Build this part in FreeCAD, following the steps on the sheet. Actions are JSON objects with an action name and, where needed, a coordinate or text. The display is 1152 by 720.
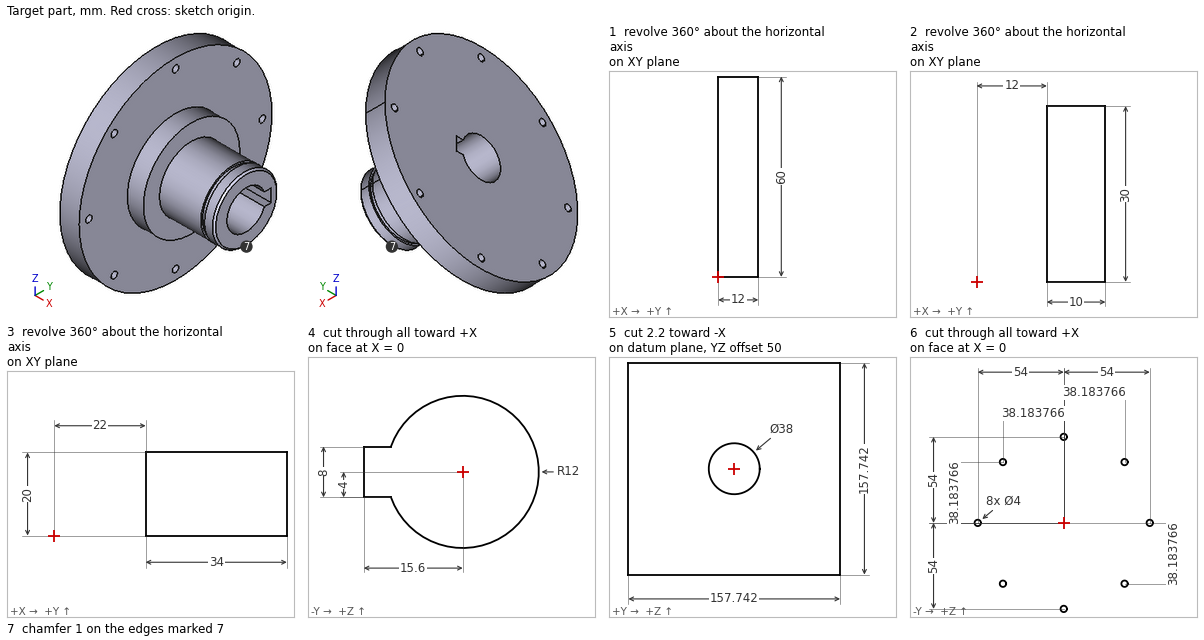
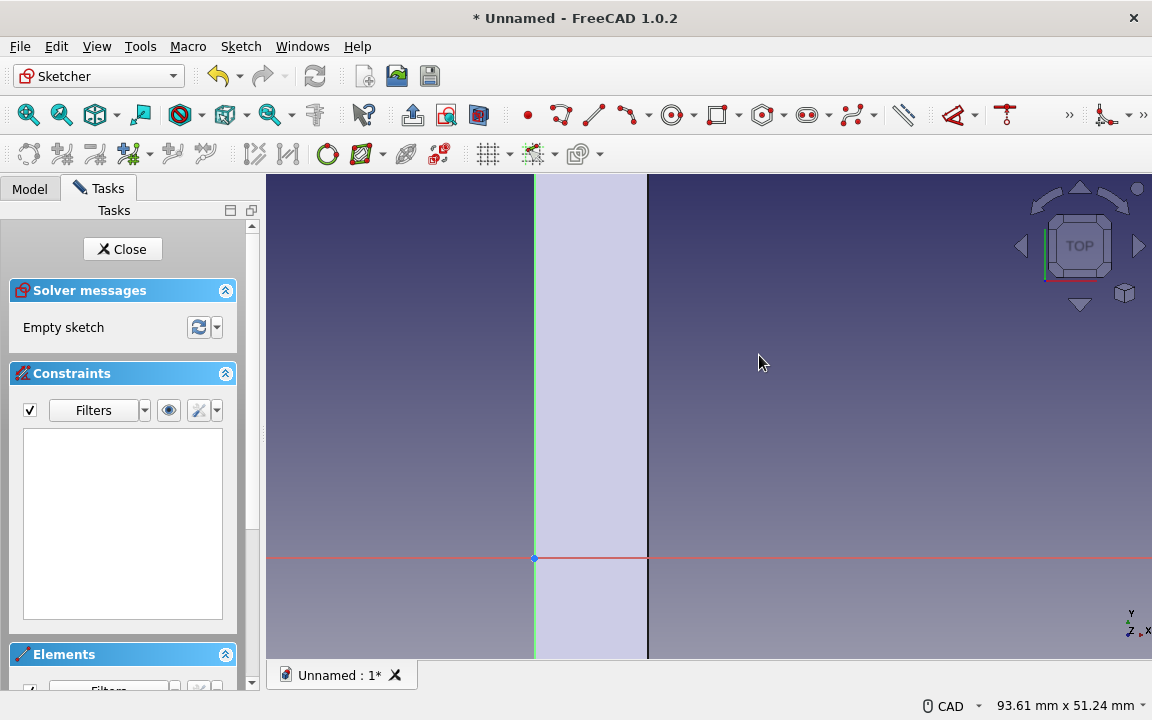
{"action": "left_click", "coordinate": [716, 116]}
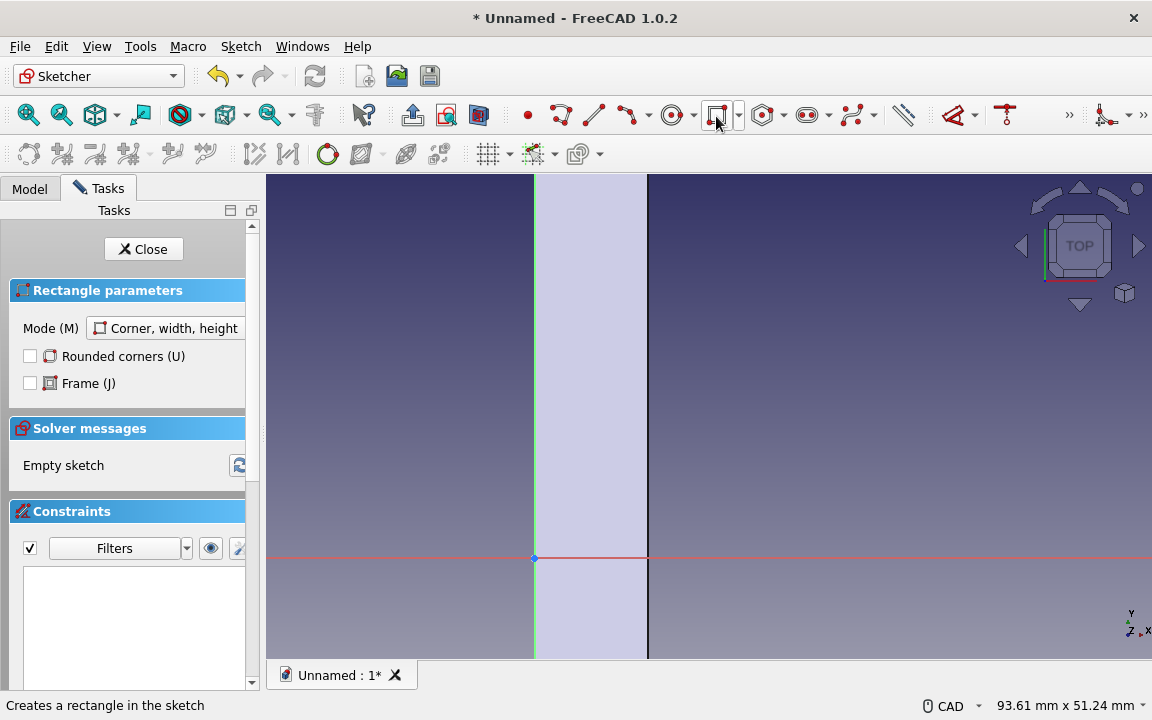
{"action": "left_click", "coordinate": [648, 274]}
{"action": "left_click", "coordinate": [743, 558]}
{"action": "key", "text": "Escape"}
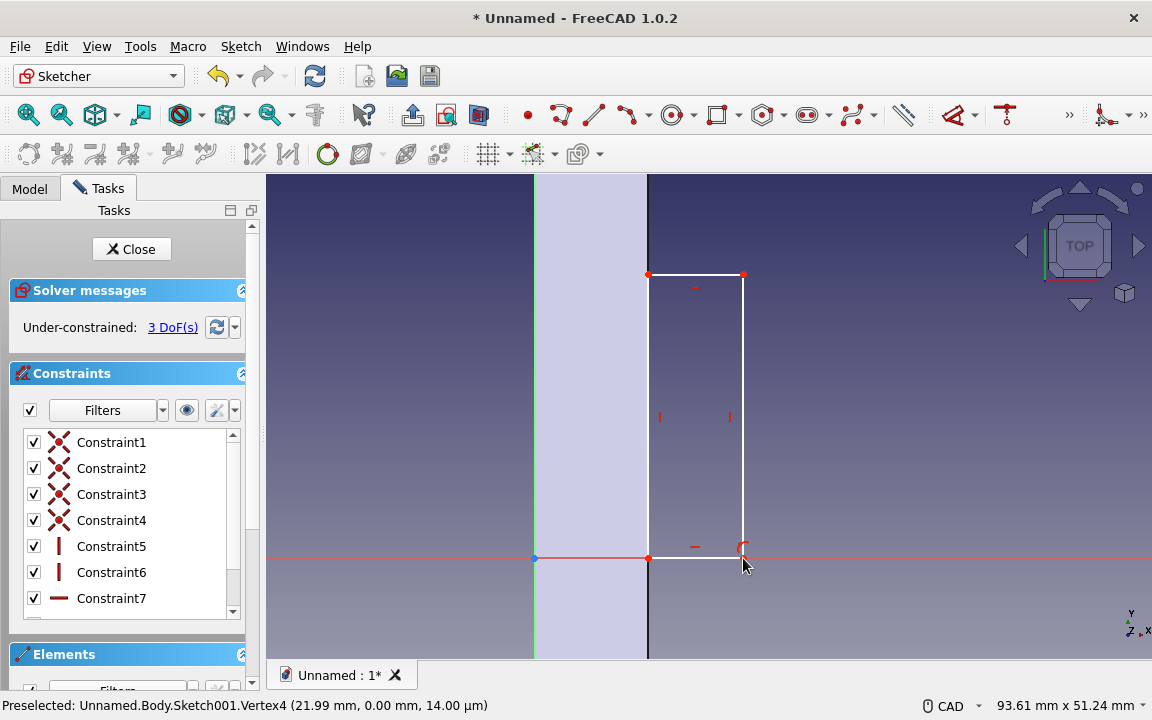
{"action": "left_click", "coordinate": [952, 116]}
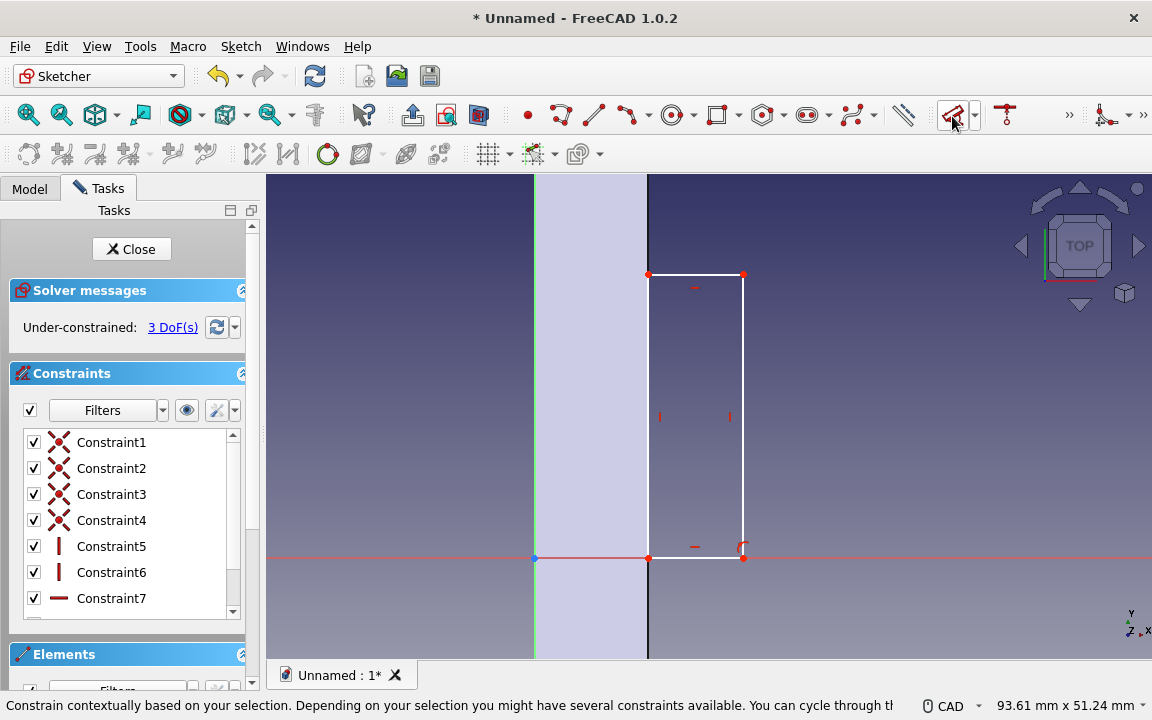
{"action": "left_click", "coordinate": [648, 360]}
{"action": "left_click", "coordinate": [682, 417]}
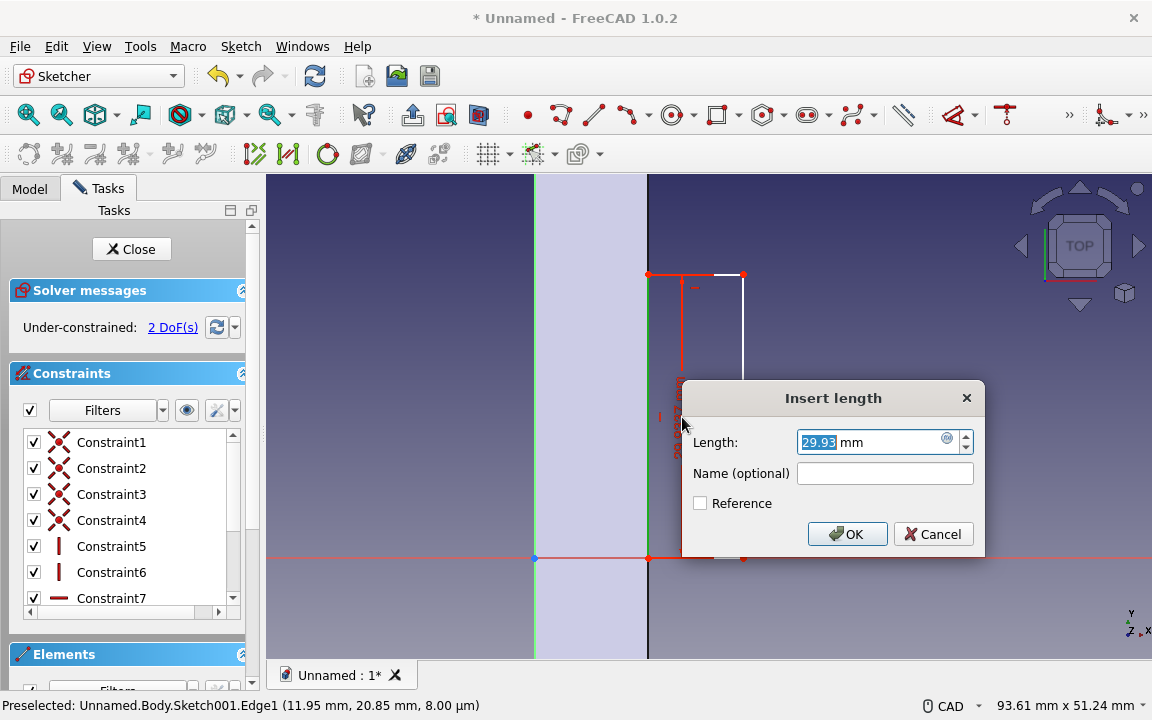
{"action": "type", "text": "30"}
{"action": "key", "text": "Return"}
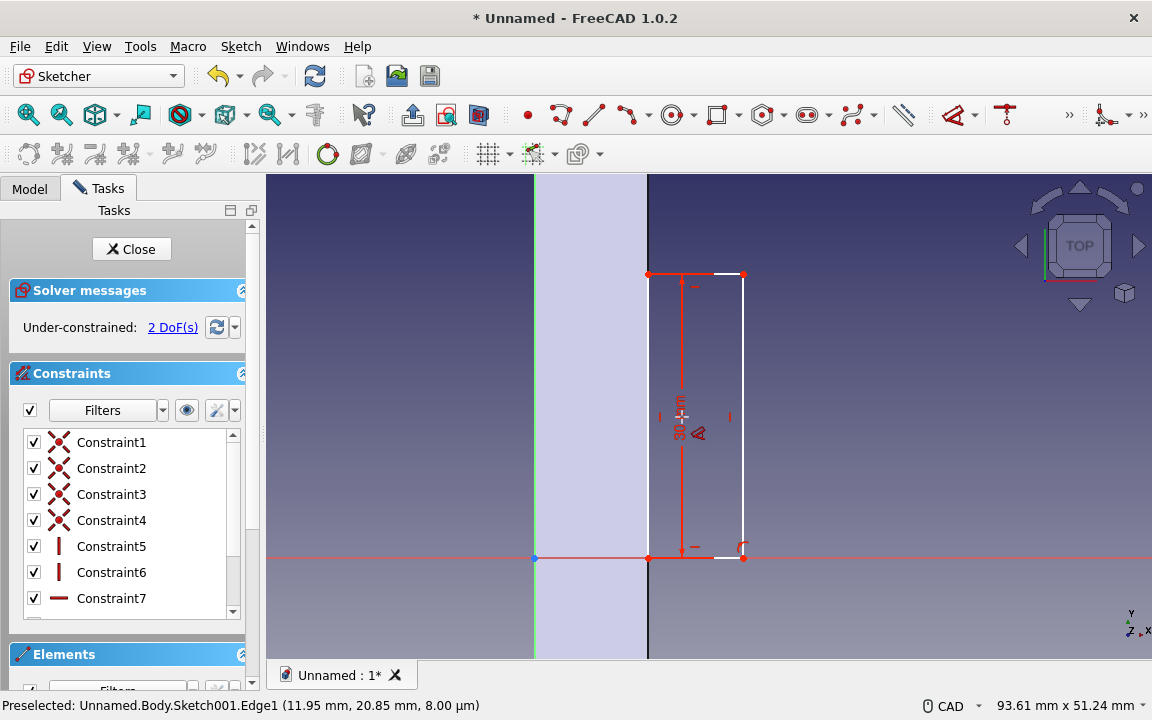
{"action": "left_click", "coordinate": [677, 558]}
{"action": "left_click", "coordinate": [696, 592]}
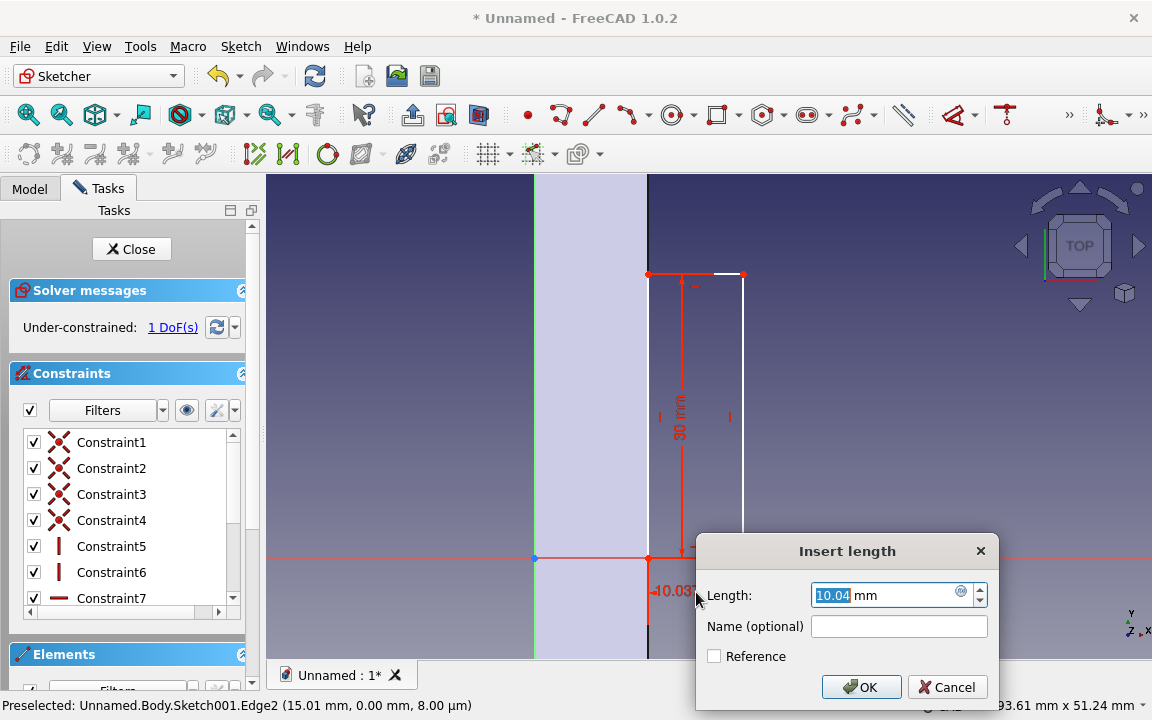
{"action": "type", "text": "10"}
{"action": "key", "text": "Return"}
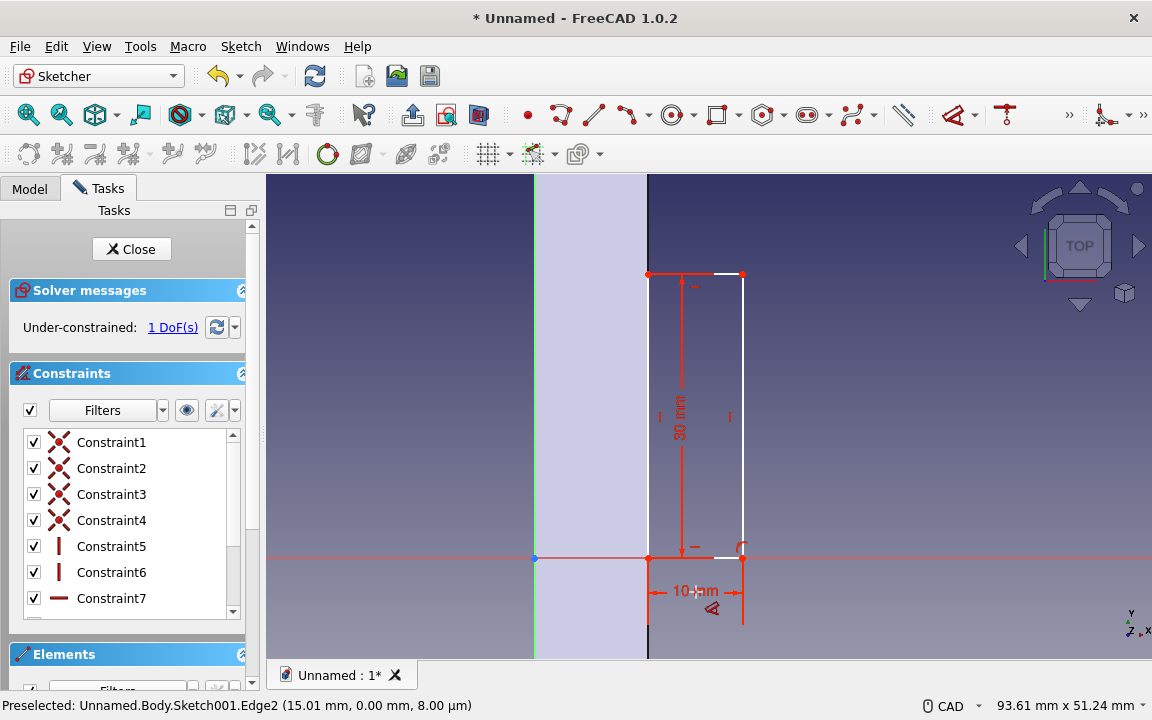
{"action": "left_click", "coordinate": [648, 274]}
{"action": "left_click", "coordinate": [591, 592]}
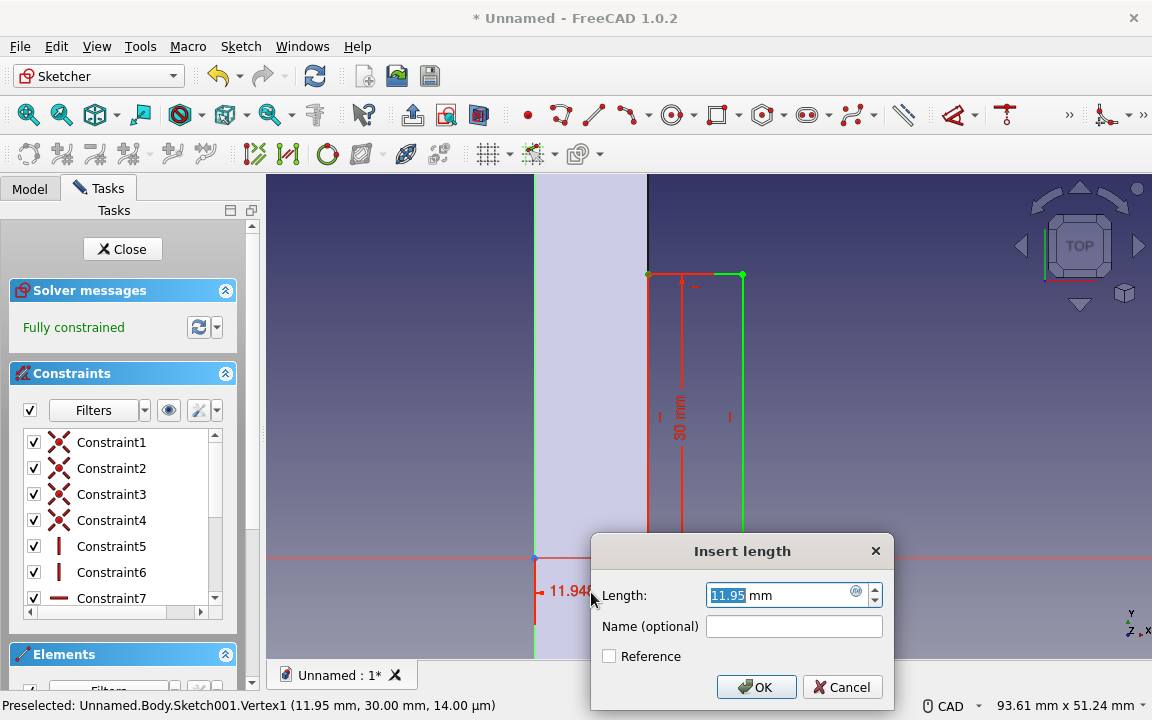
{"action": "type", "text": "12"}
{"action": "key", "text": "Return"}
{"action": "key", "text": "Escape"}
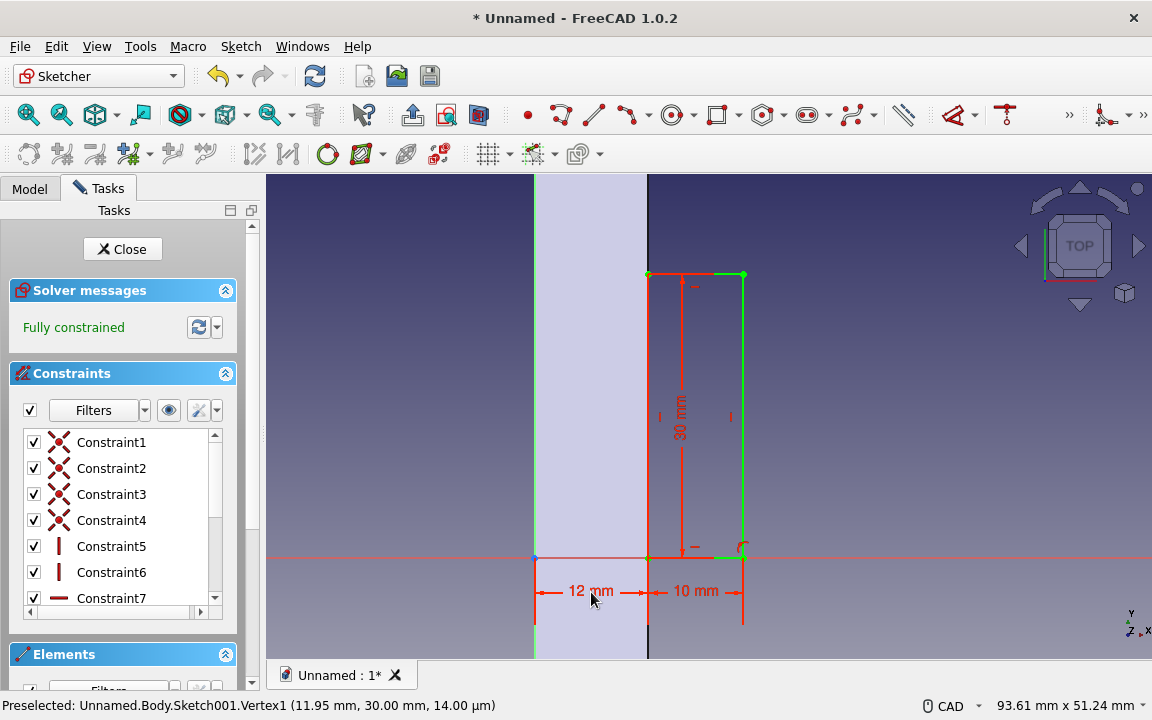
{"action": "left_click", "coordinate": [123, 249]}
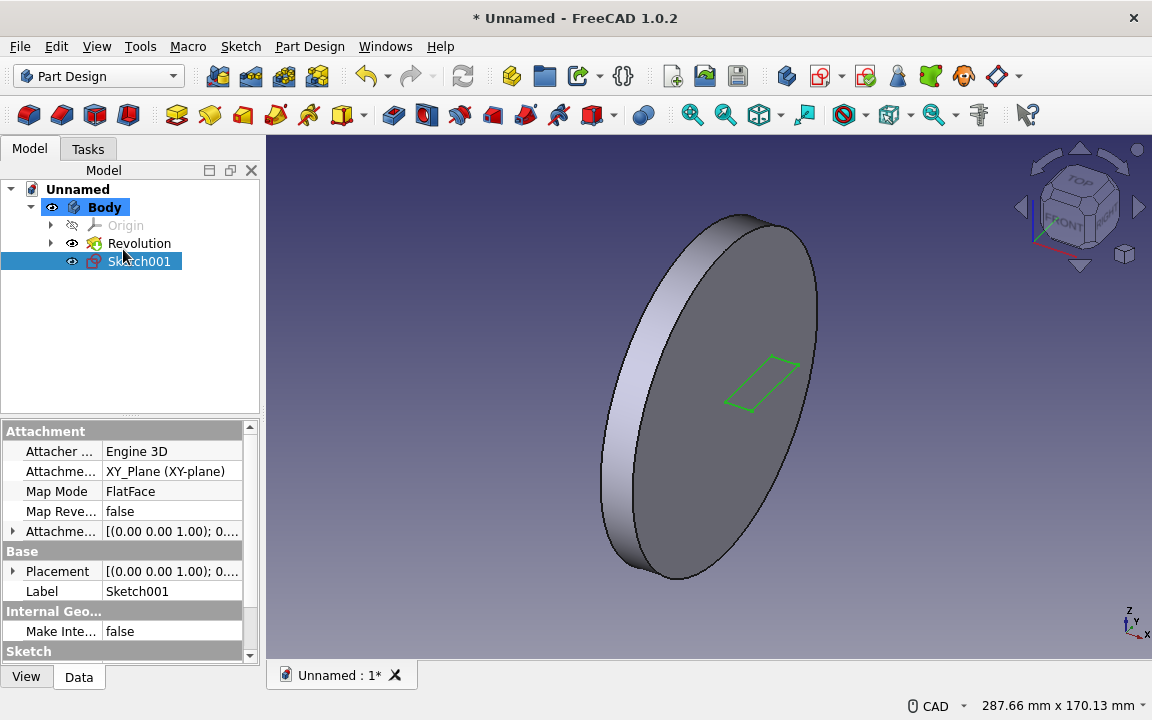
{"action": "left_click", "coordinate": [210, 116]}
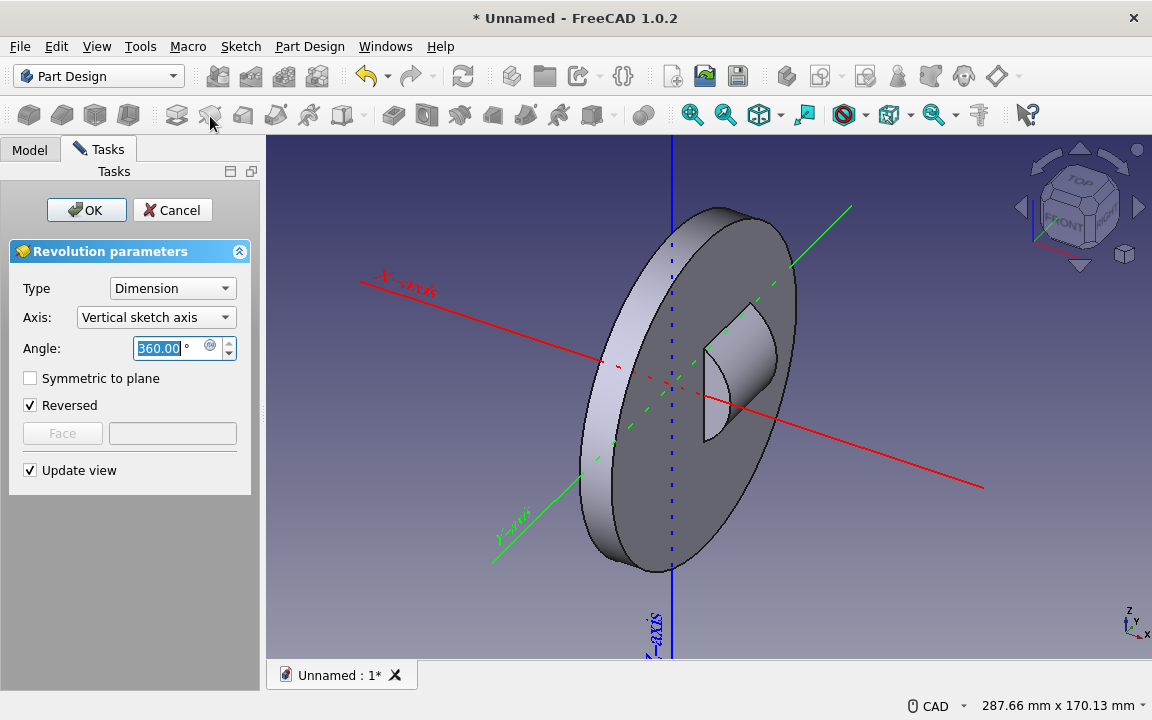
{"action": "left_click", "coordinate": [157, 318]}